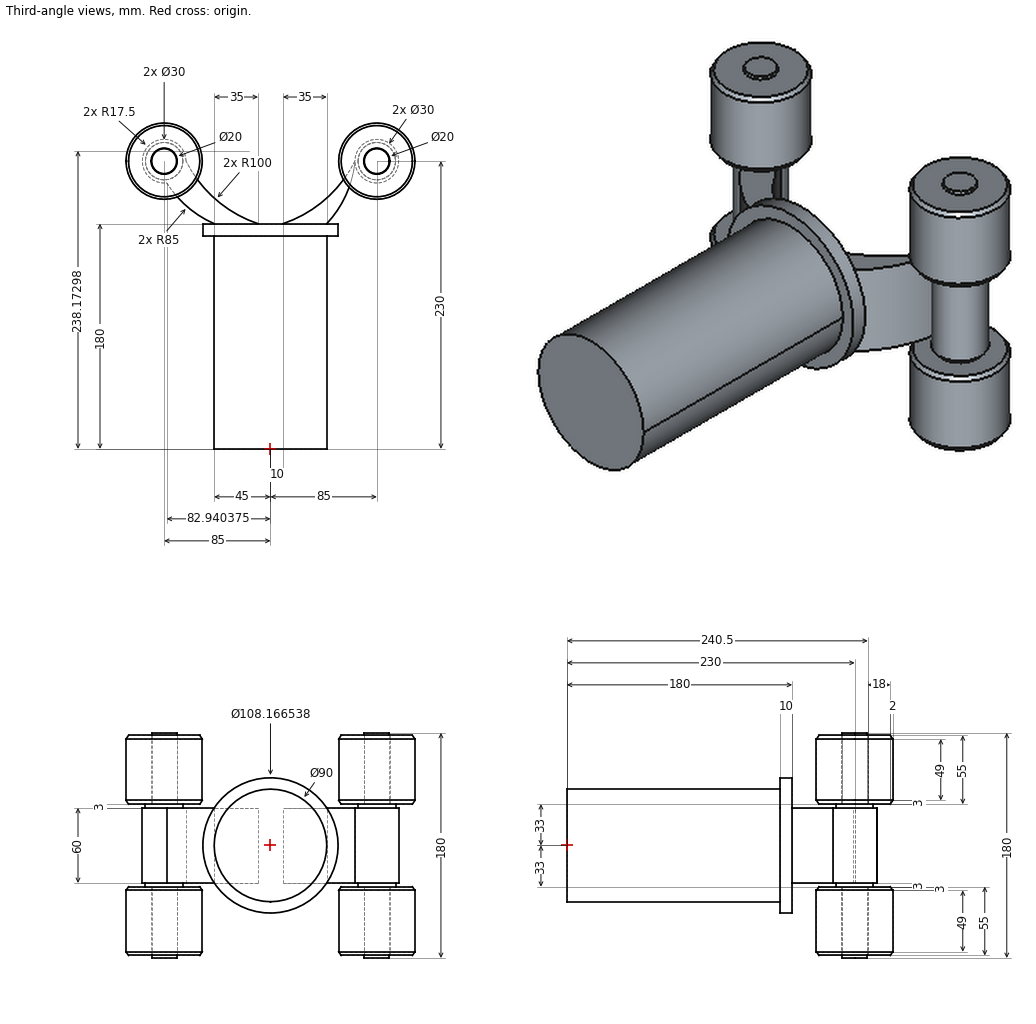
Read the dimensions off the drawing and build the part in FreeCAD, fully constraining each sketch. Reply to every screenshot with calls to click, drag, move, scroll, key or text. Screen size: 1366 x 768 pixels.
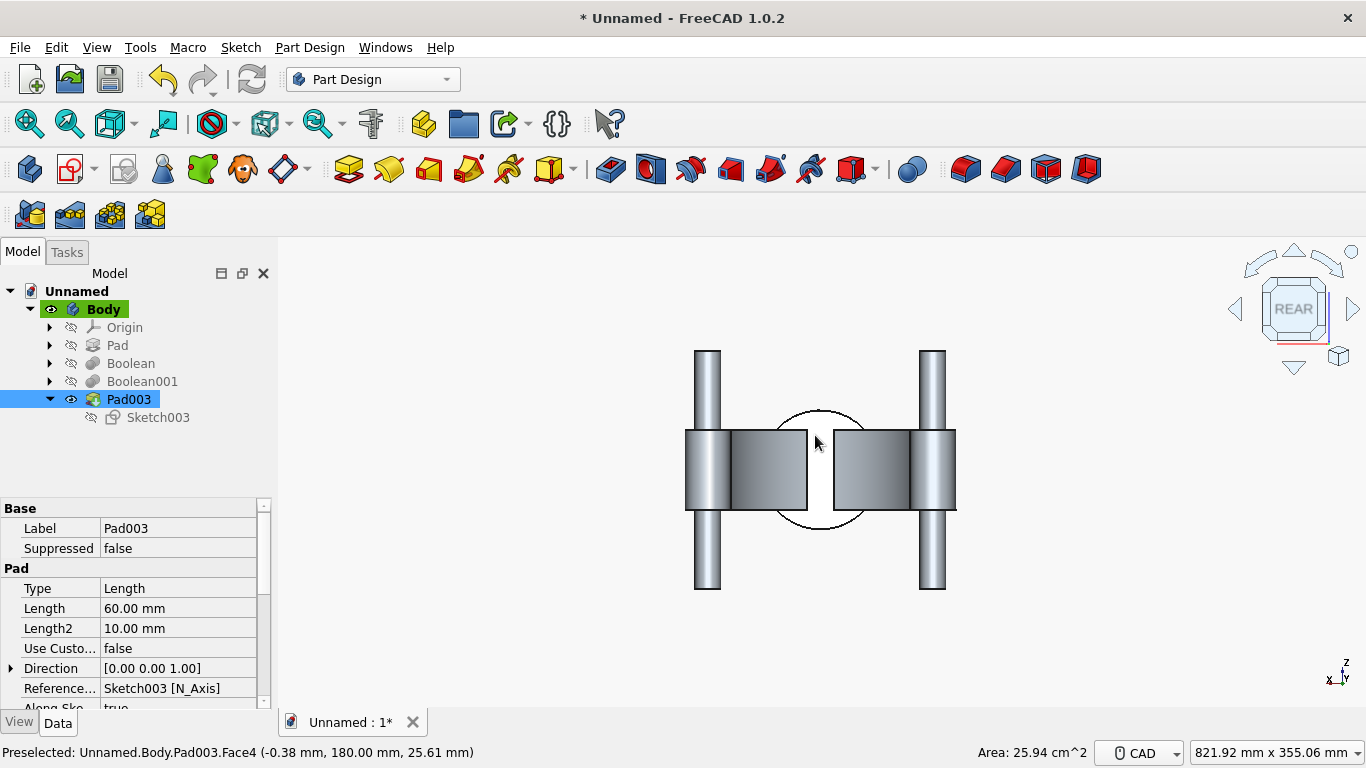
click(70, 170)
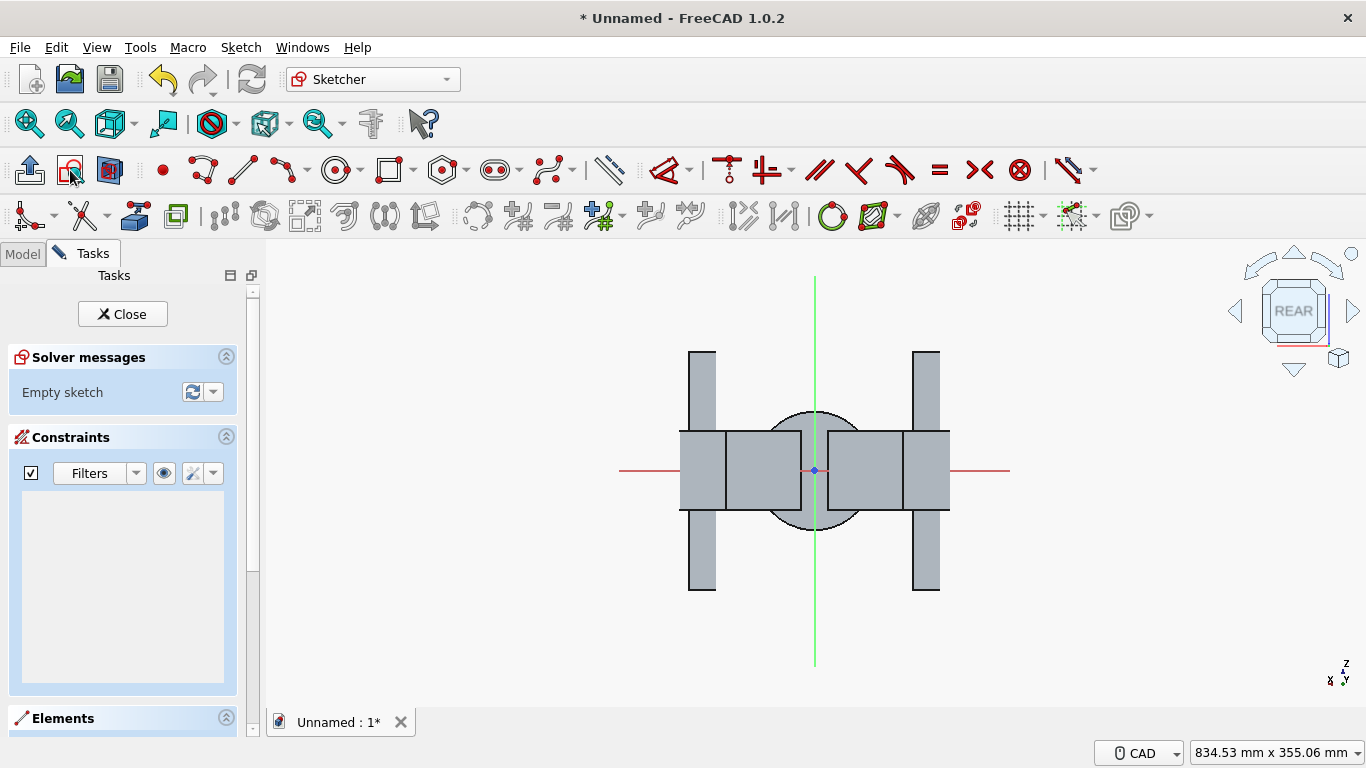
scroll(869, 469, up, 4)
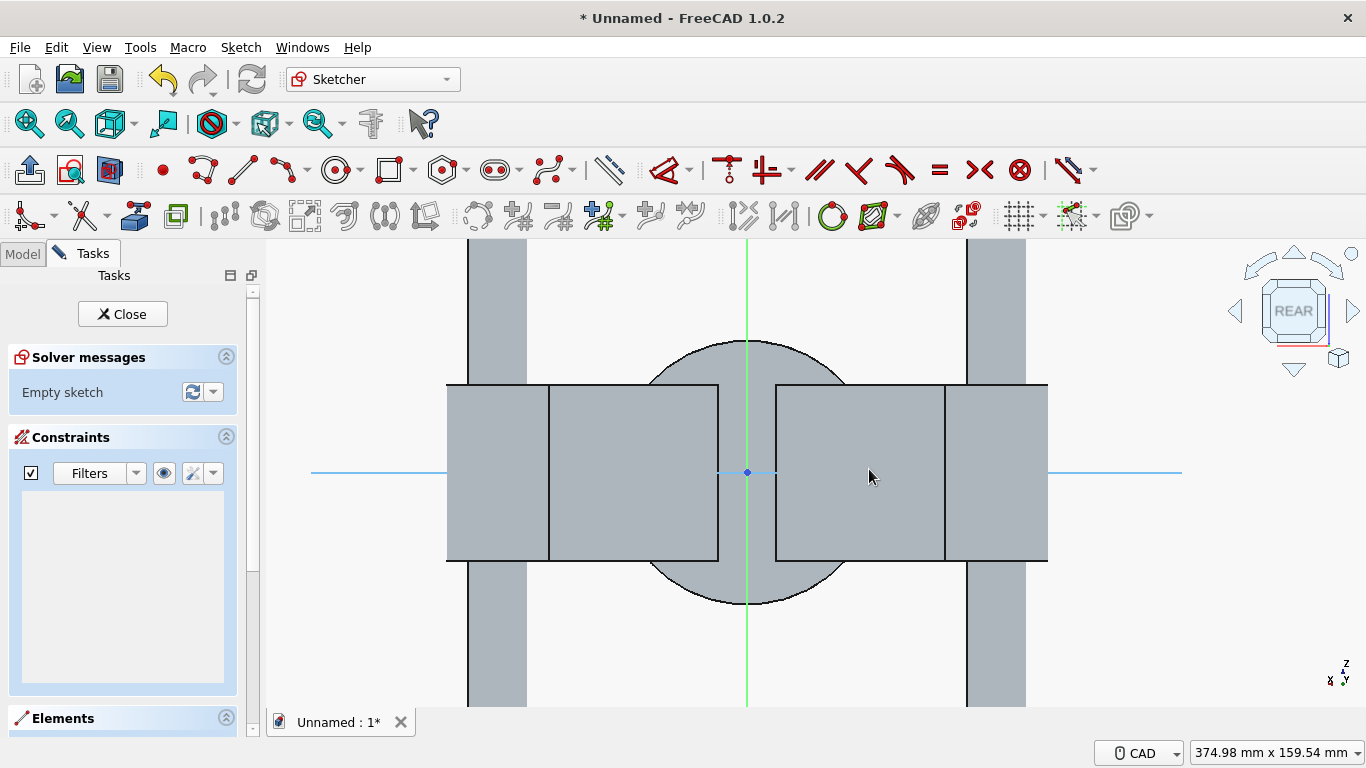
click(336, 170)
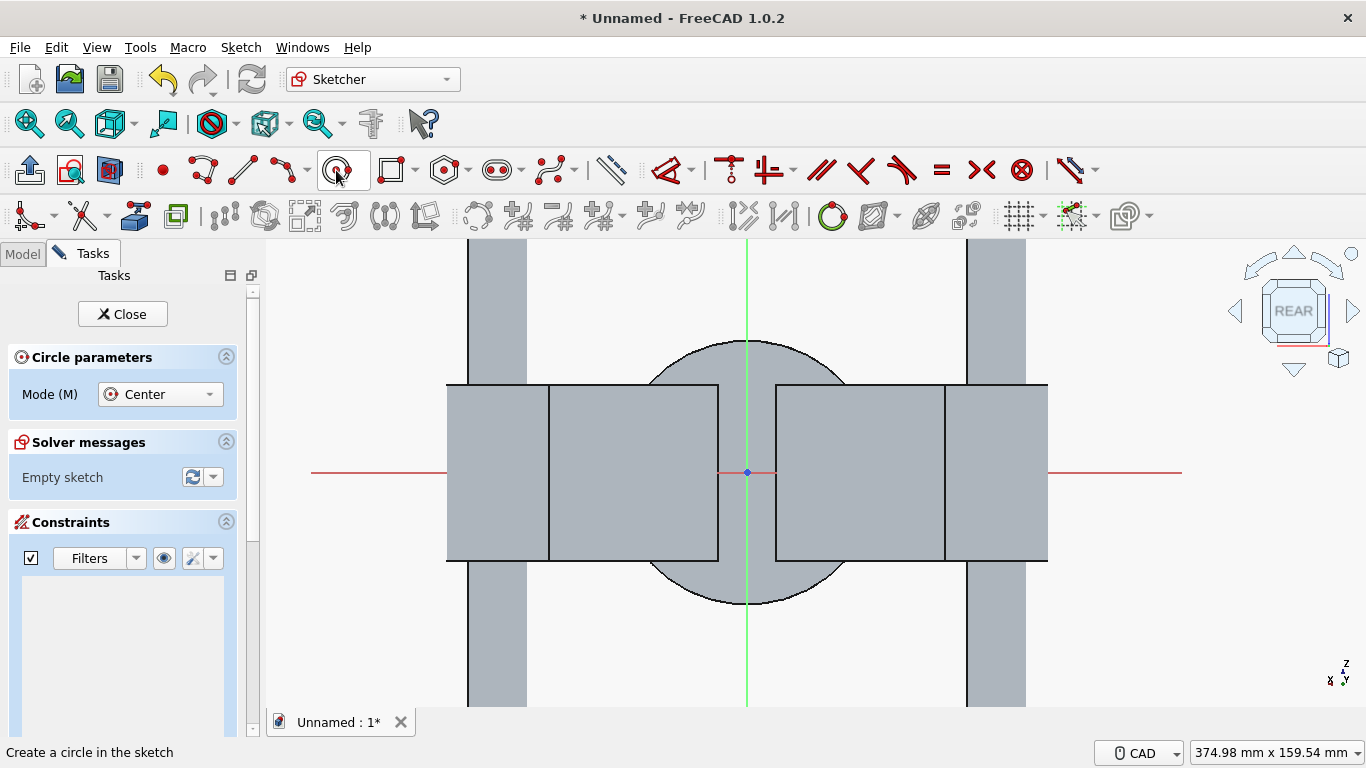
click(747, 473)
click(859, 360)
key(Escape)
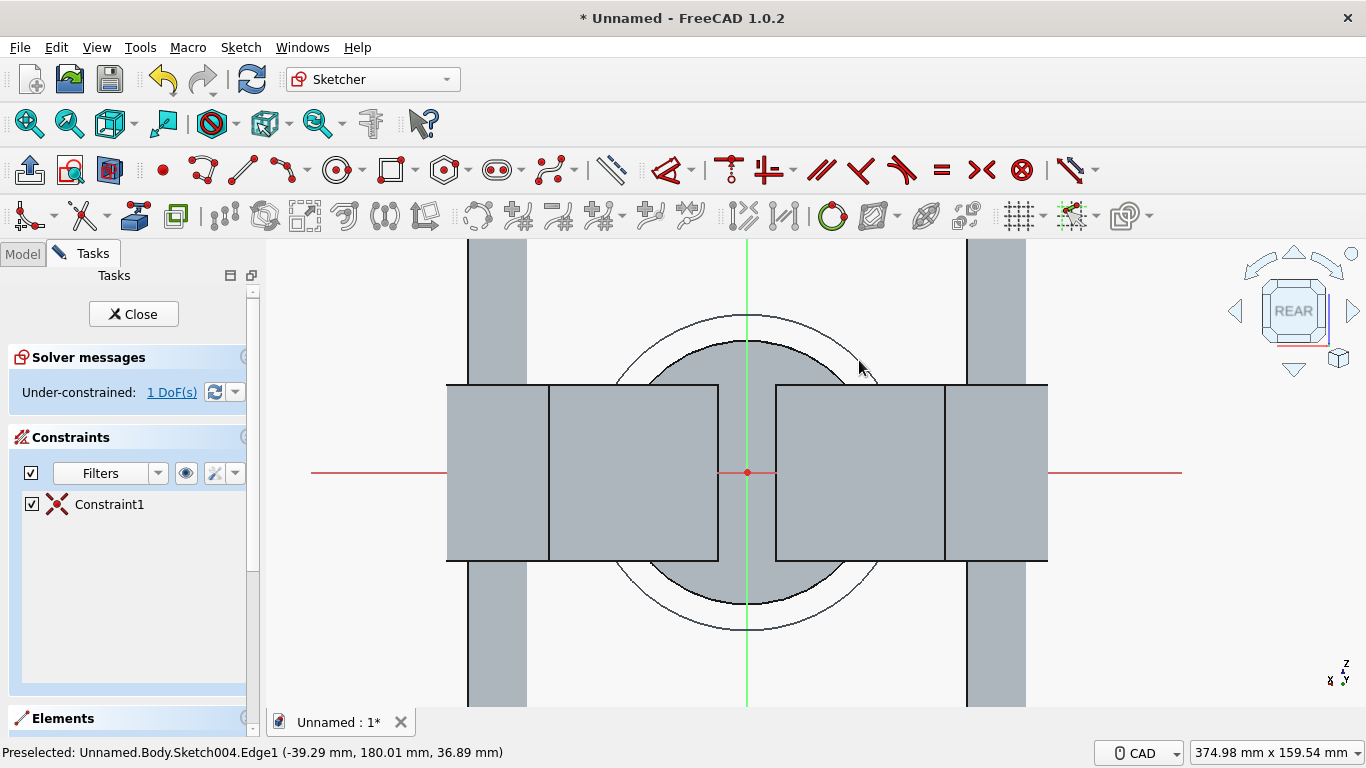
click(666, 170)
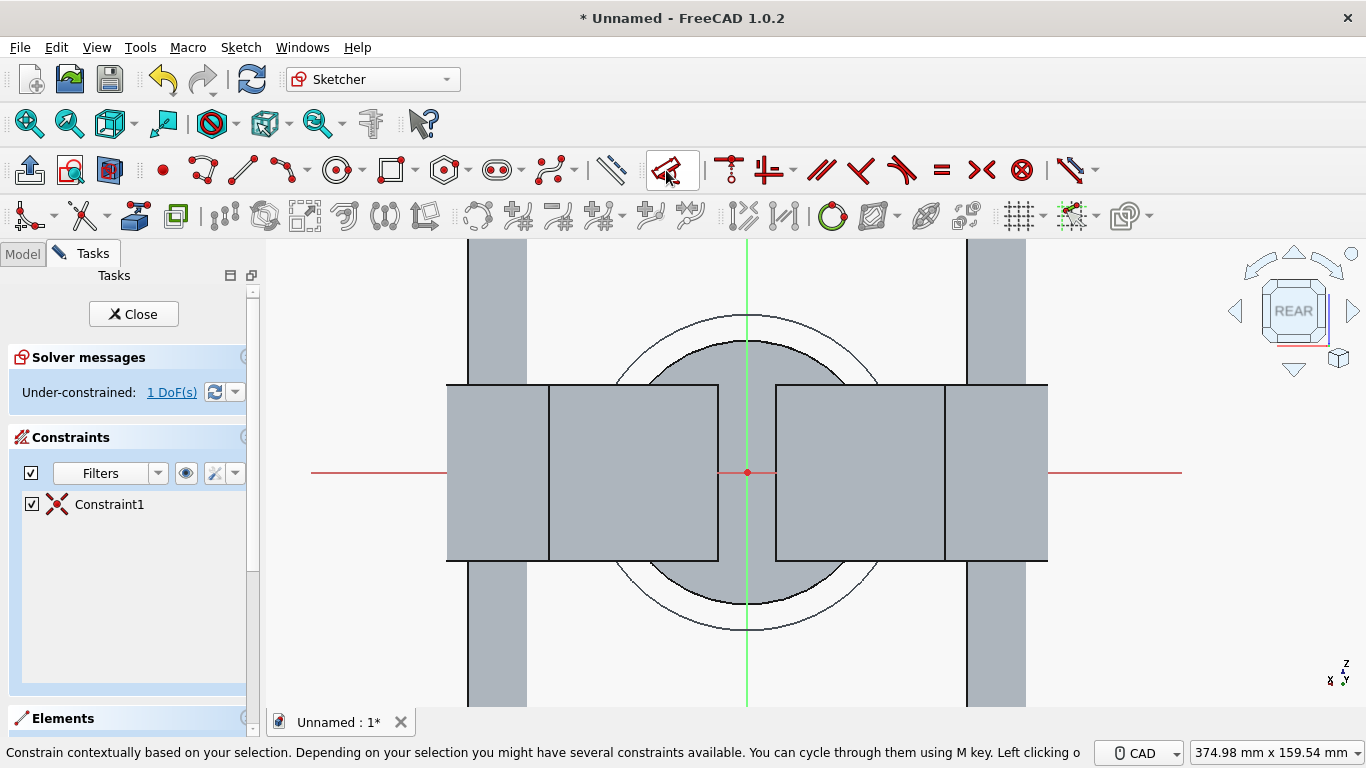
click(859, 361)
click(882, 338)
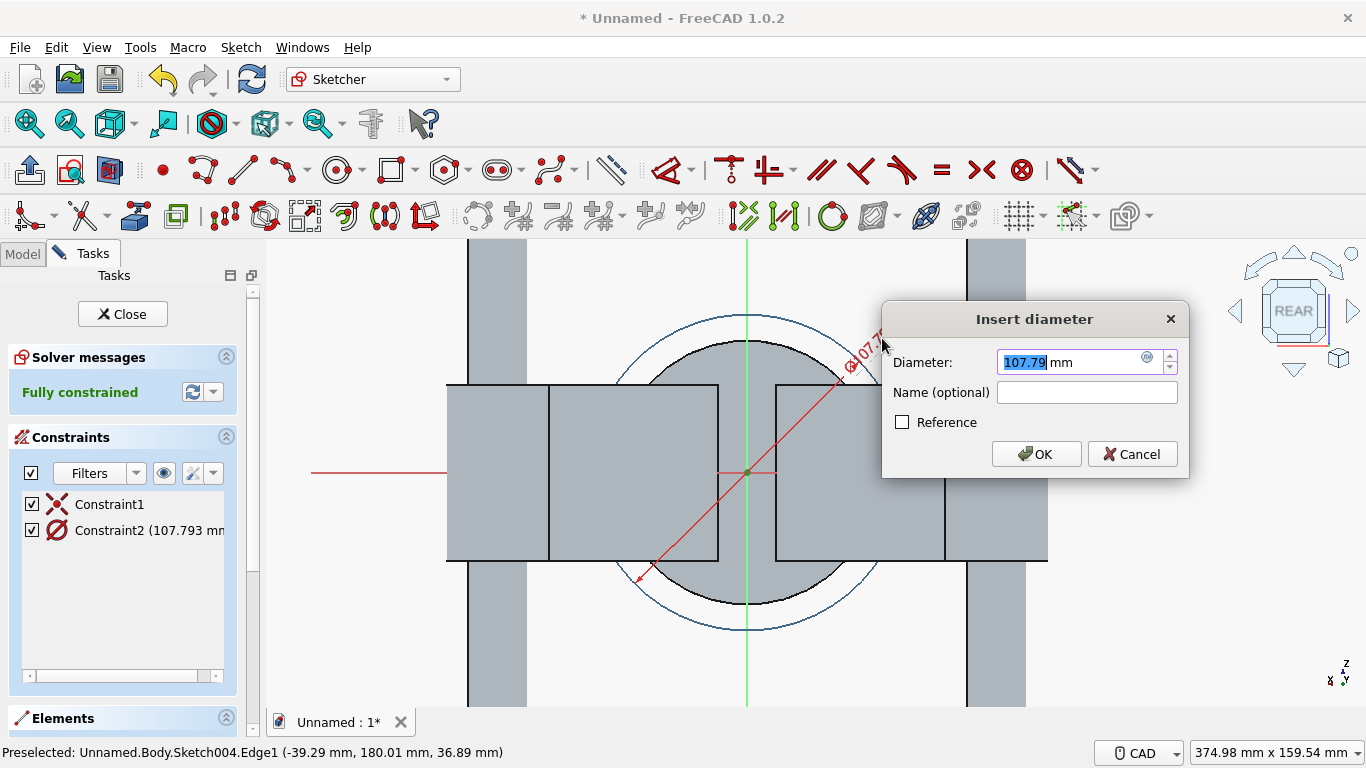
text(108.166538)
key(Return)
key(Escape)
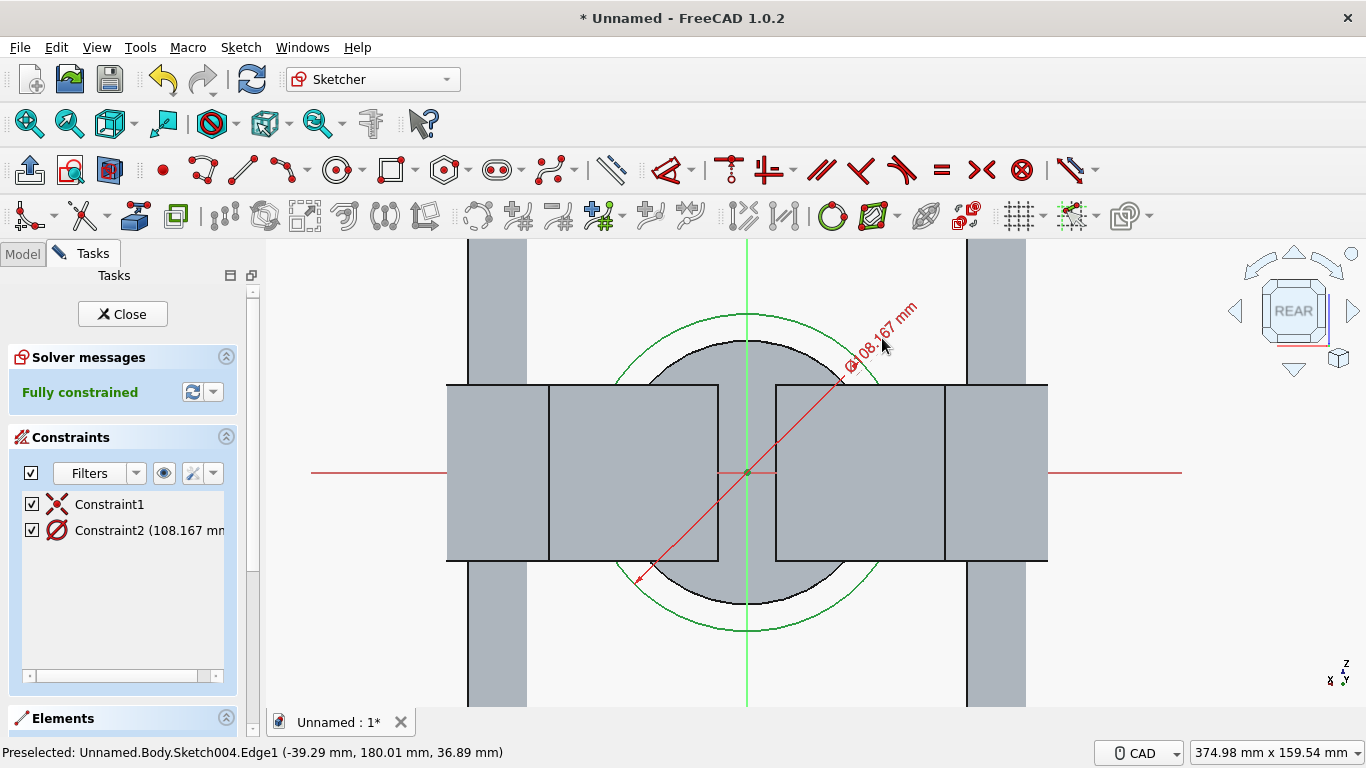
click(123, 314)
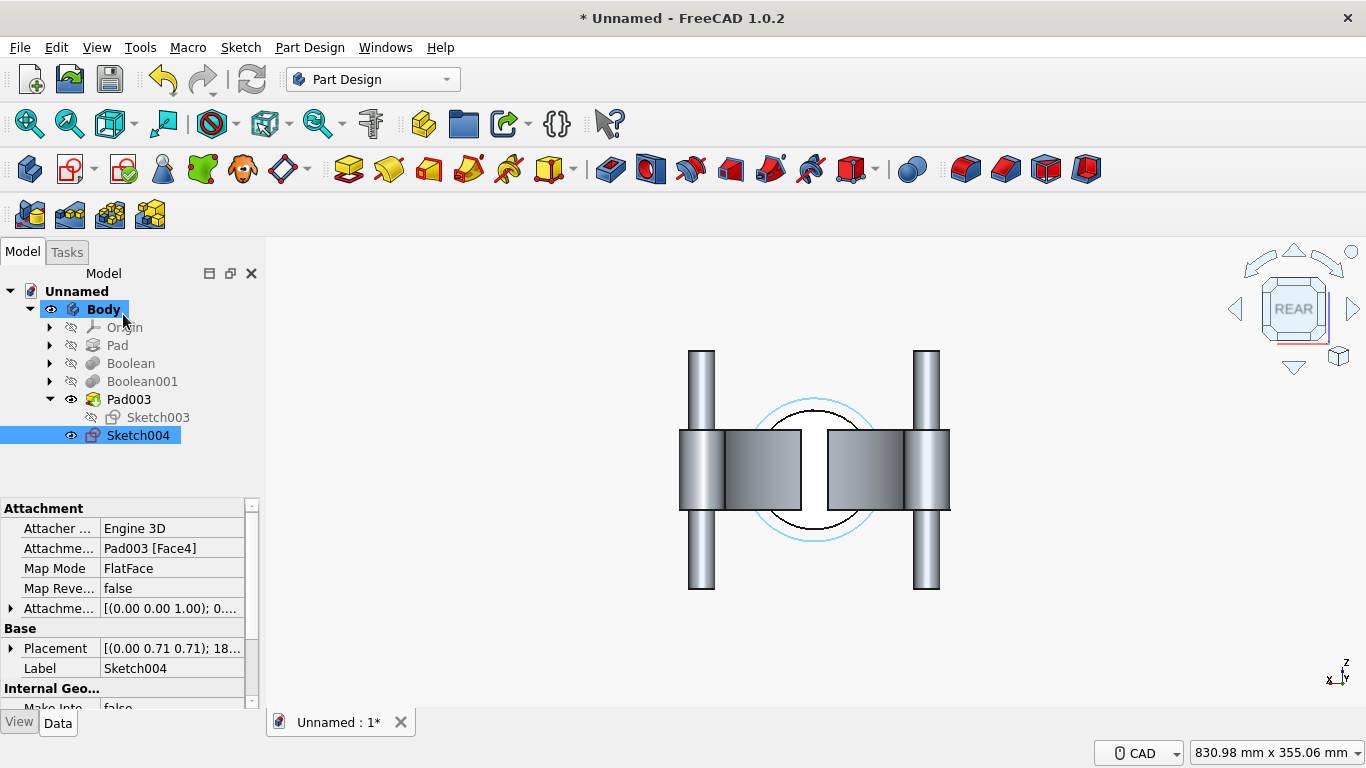
click(350, 170)